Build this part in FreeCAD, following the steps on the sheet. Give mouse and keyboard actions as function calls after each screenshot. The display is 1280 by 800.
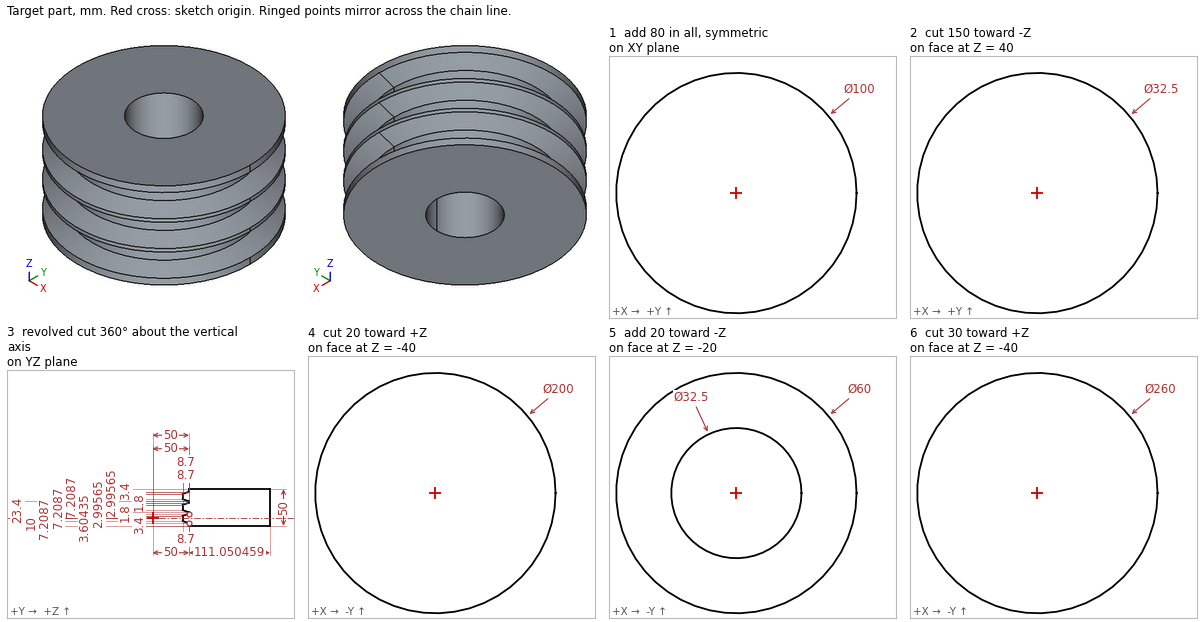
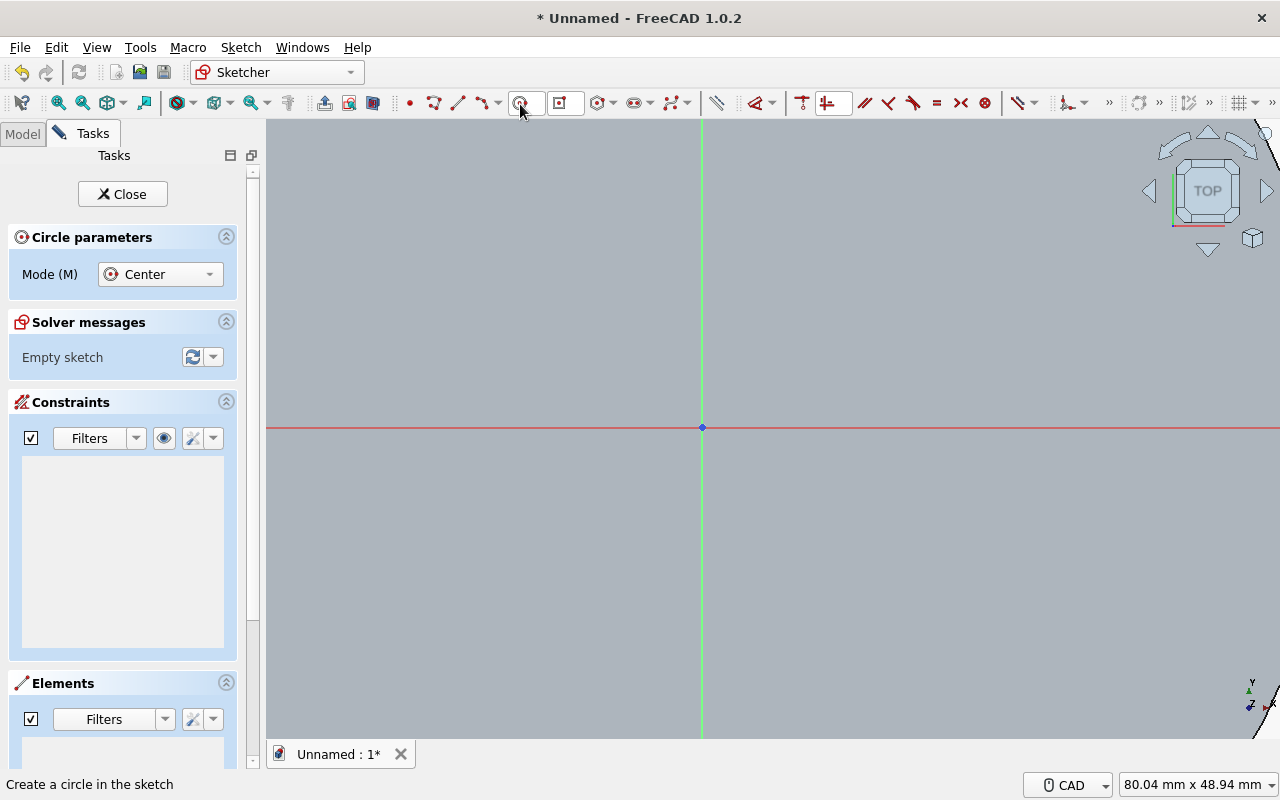
click(702, 428)
click(848, 282)
key(Escape)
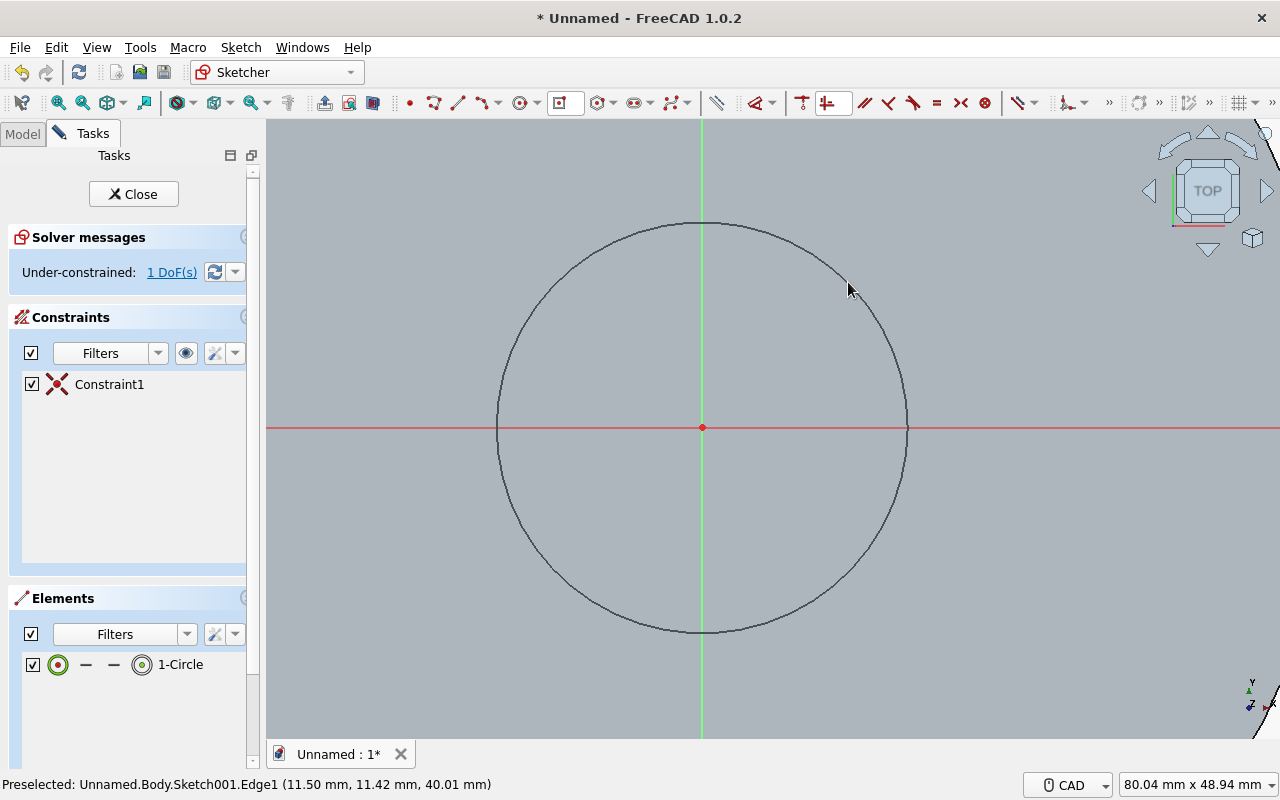
key(d)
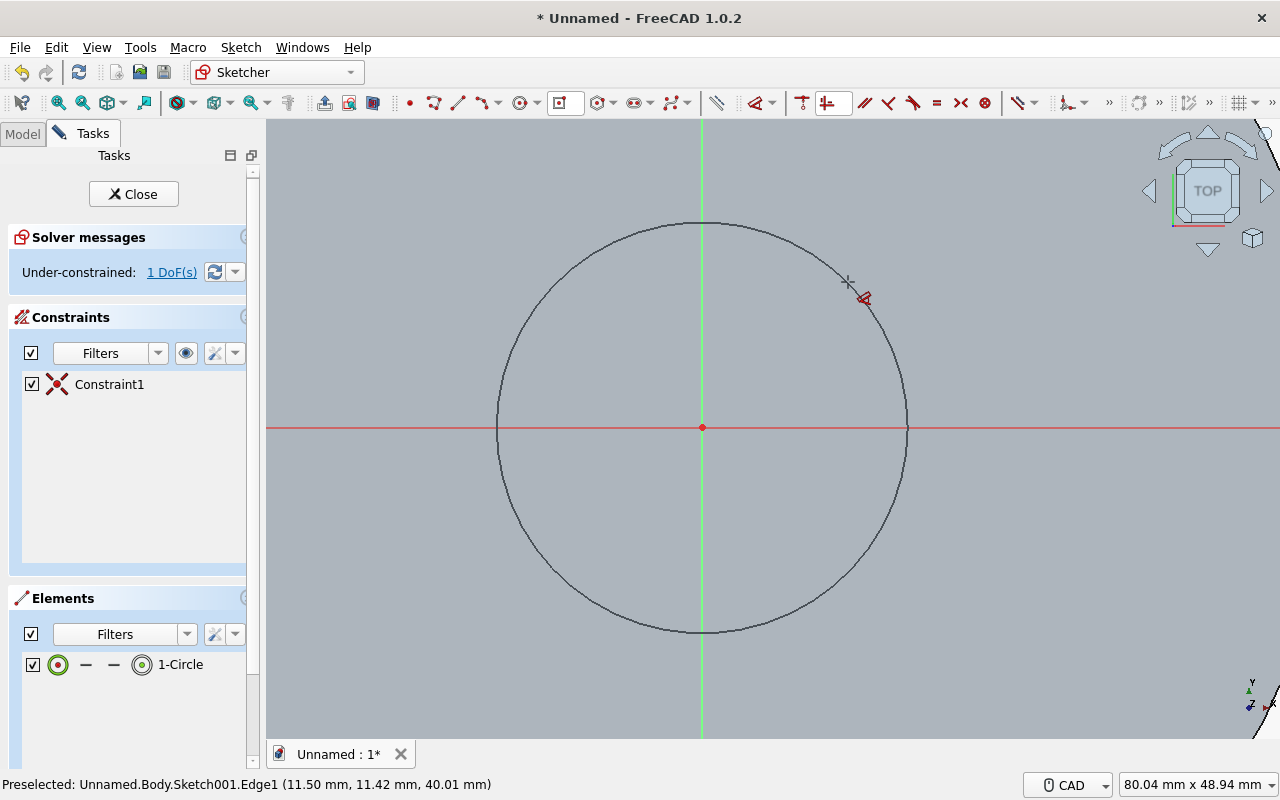
click(847, 282)
click(870, 259)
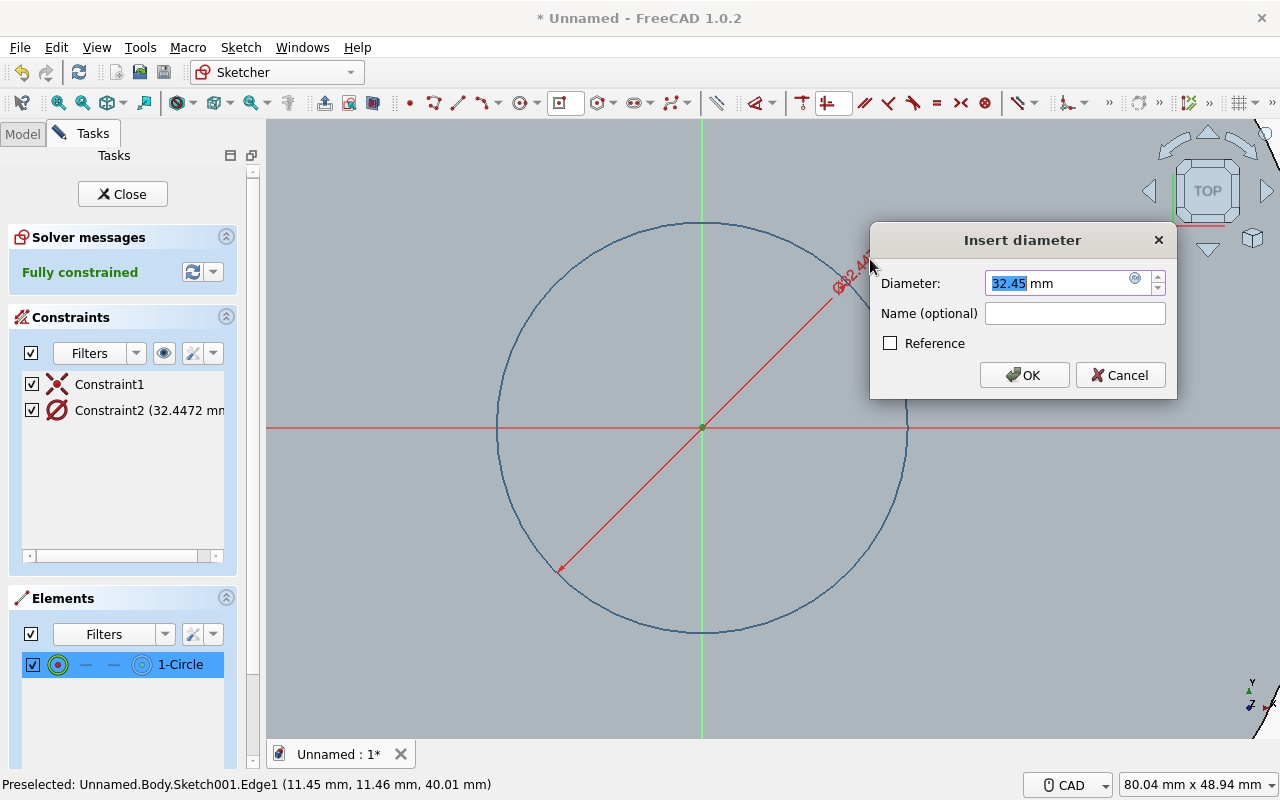
text(32.5)
key(Return)
key(Escape)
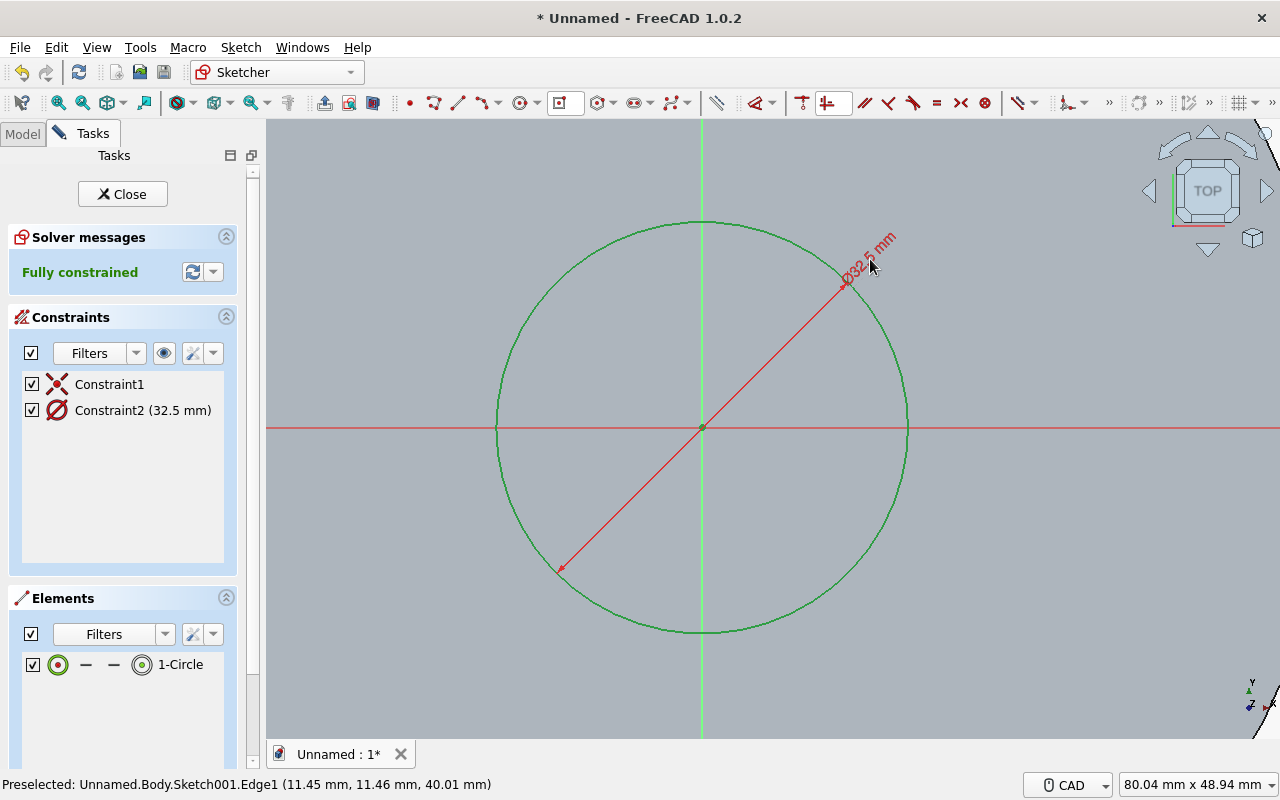
click(123, 194)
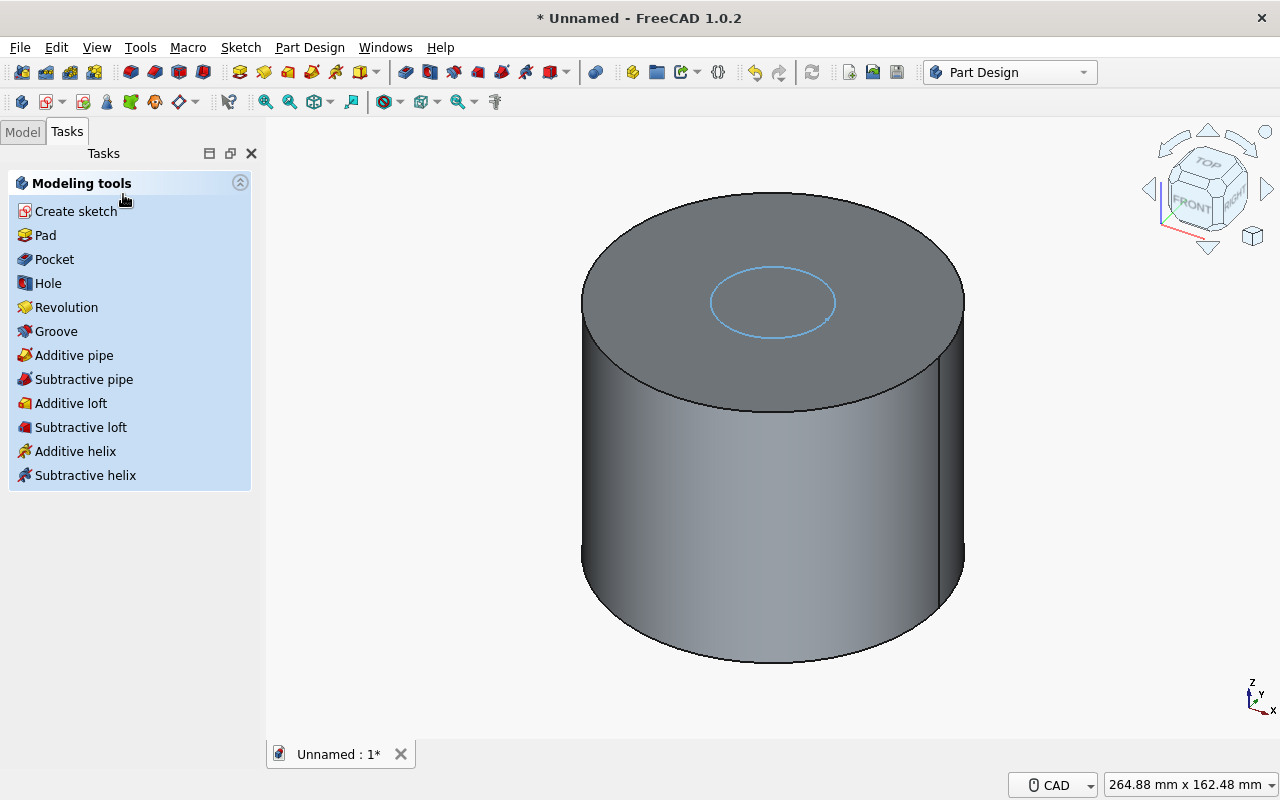
click(406, 72)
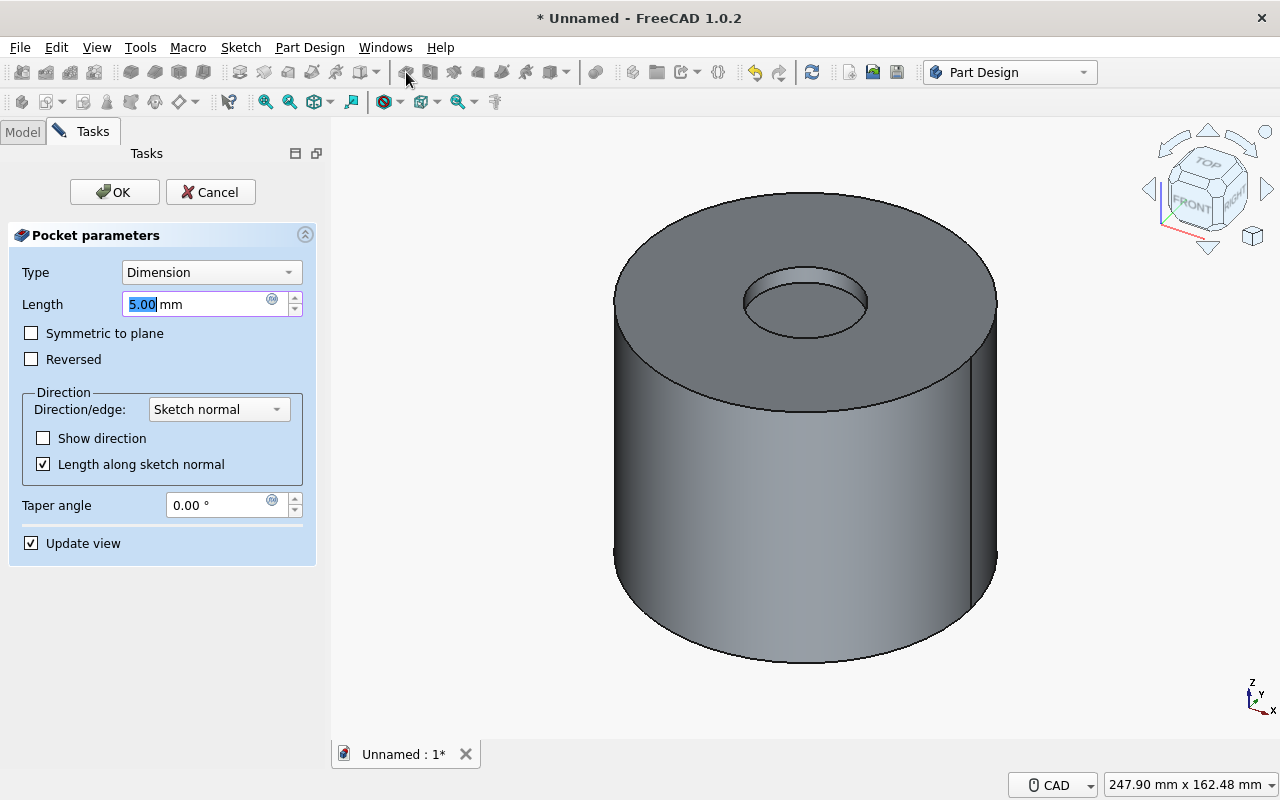
text(150)
key(Tab)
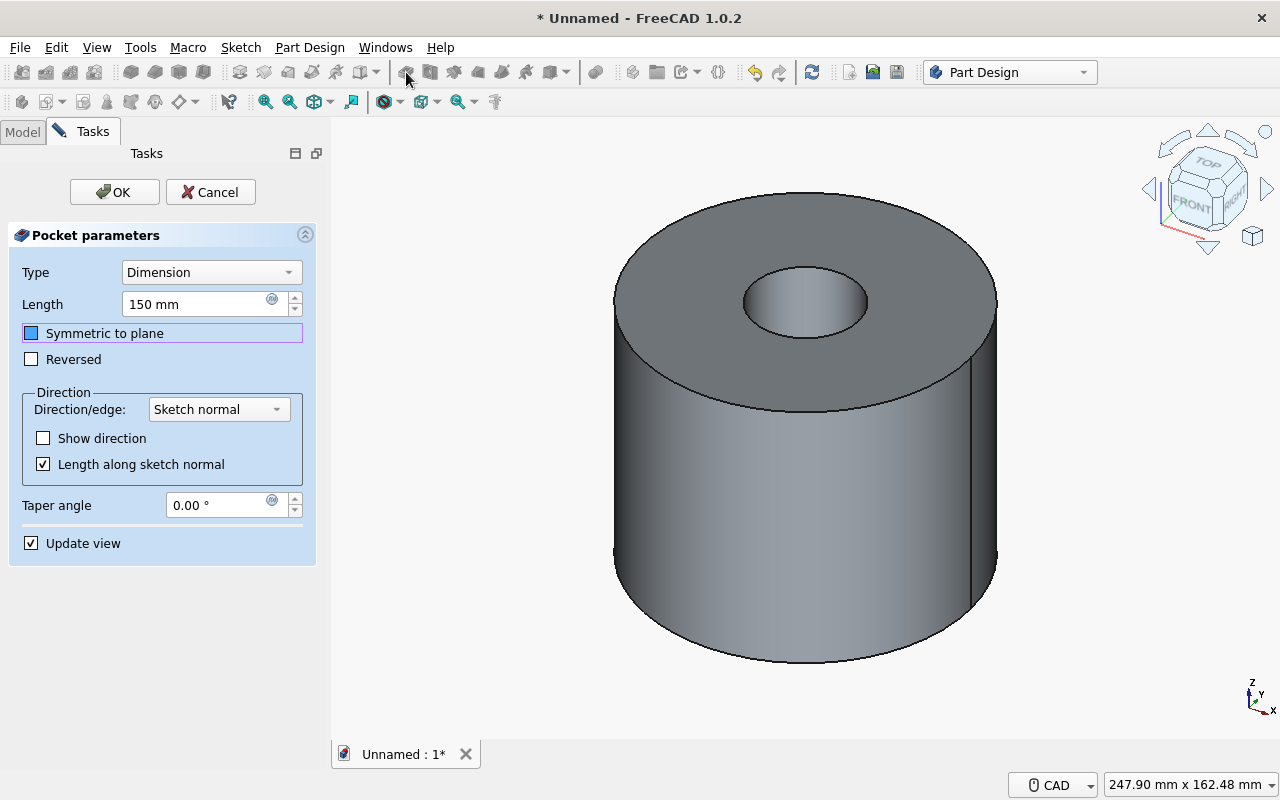
click(115, 192)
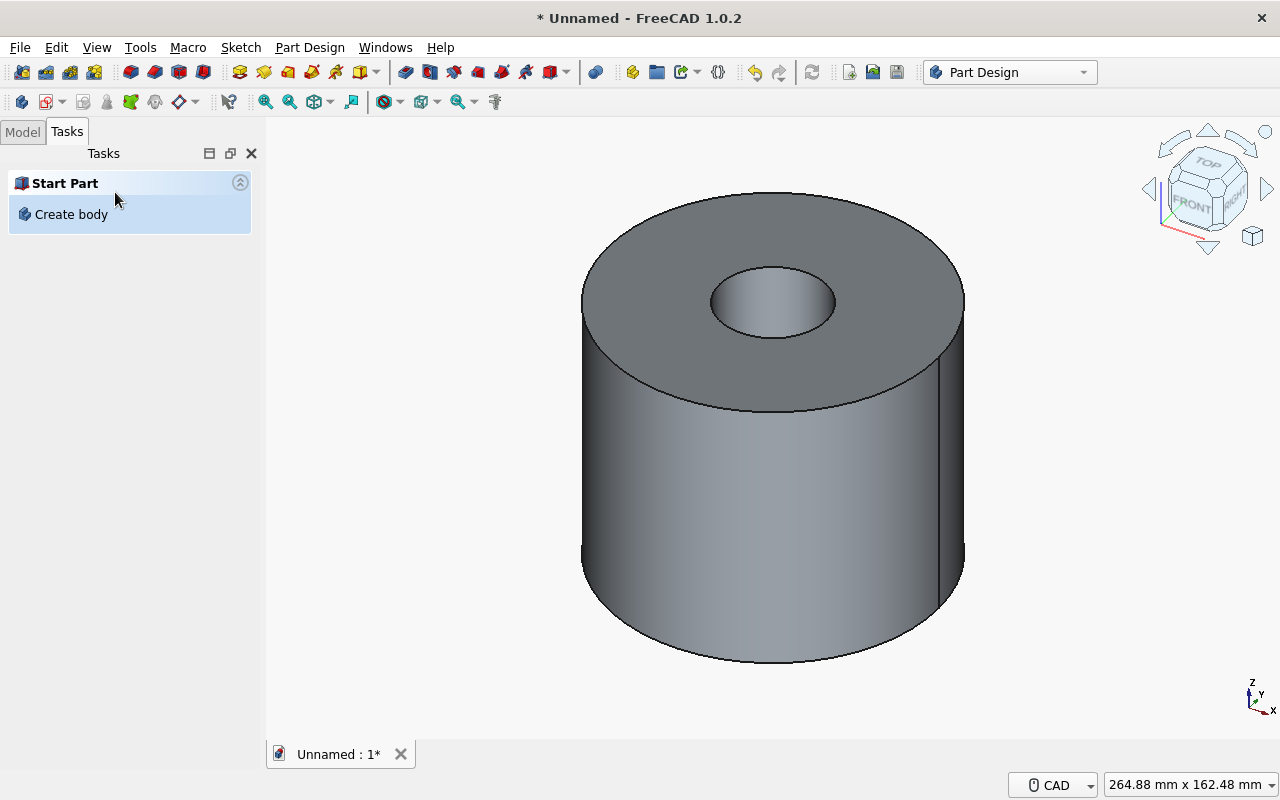
click(46, 102)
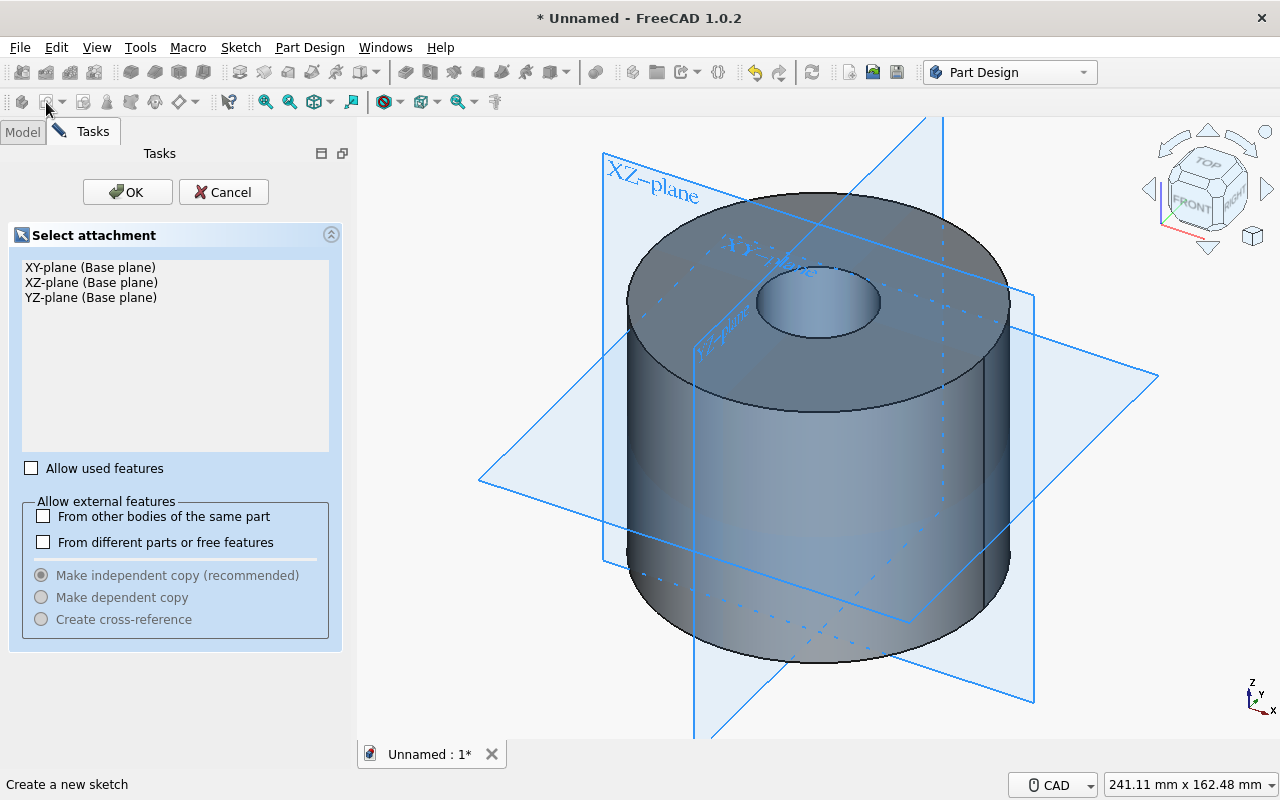
click(82, 298)